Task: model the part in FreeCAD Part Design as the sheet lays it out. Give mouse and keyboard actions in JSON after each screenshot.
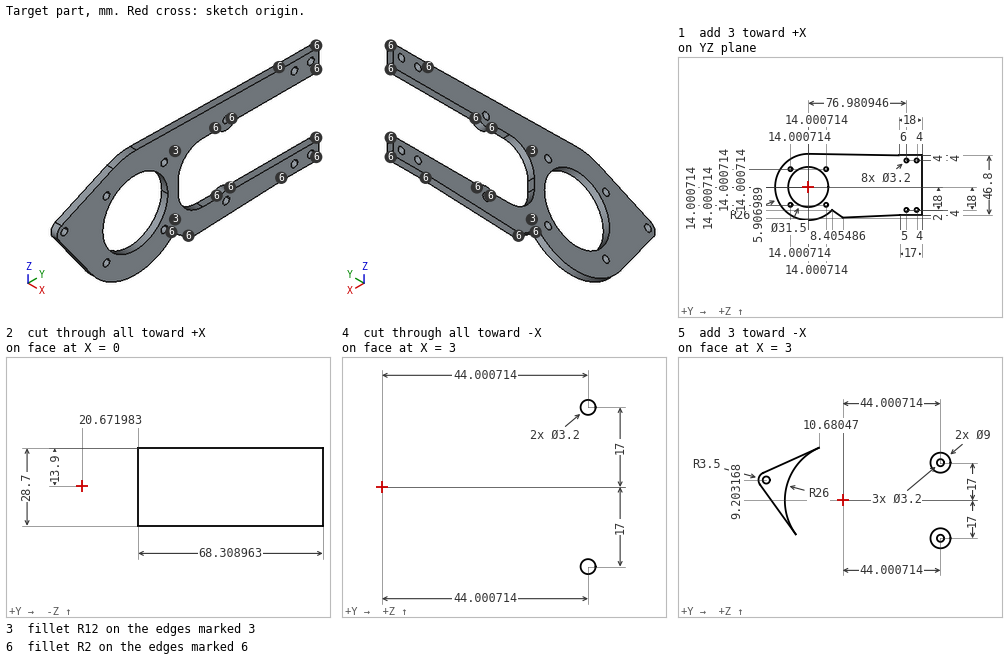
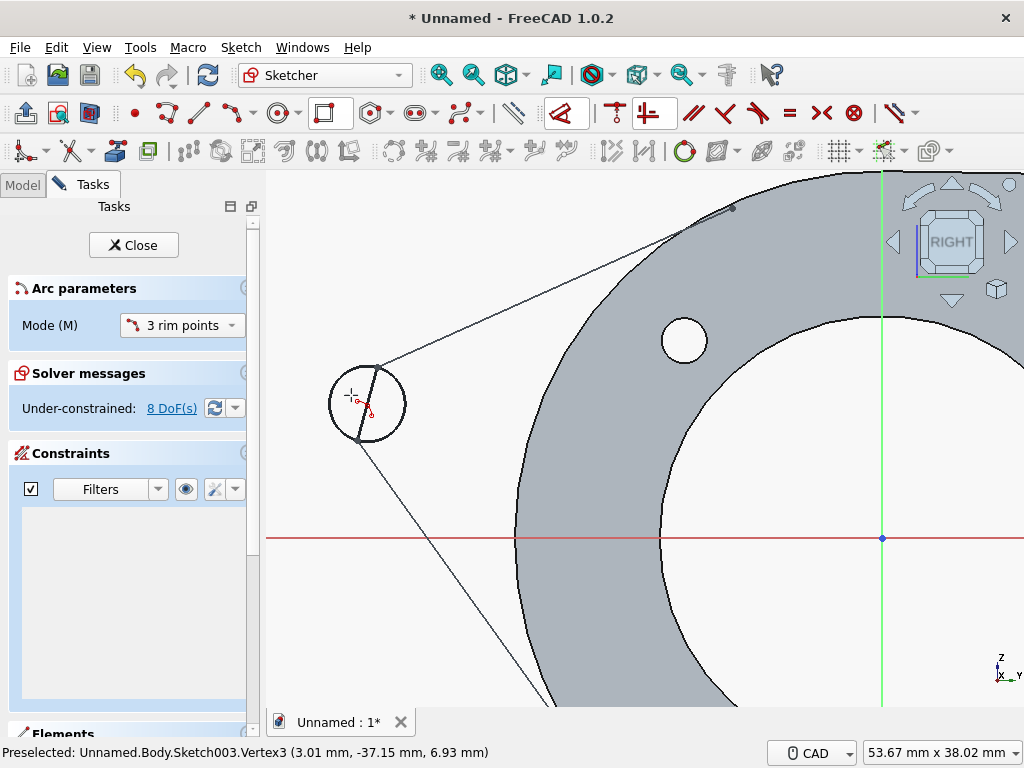
{"action": "left_click", "coordinate": [349, 396]}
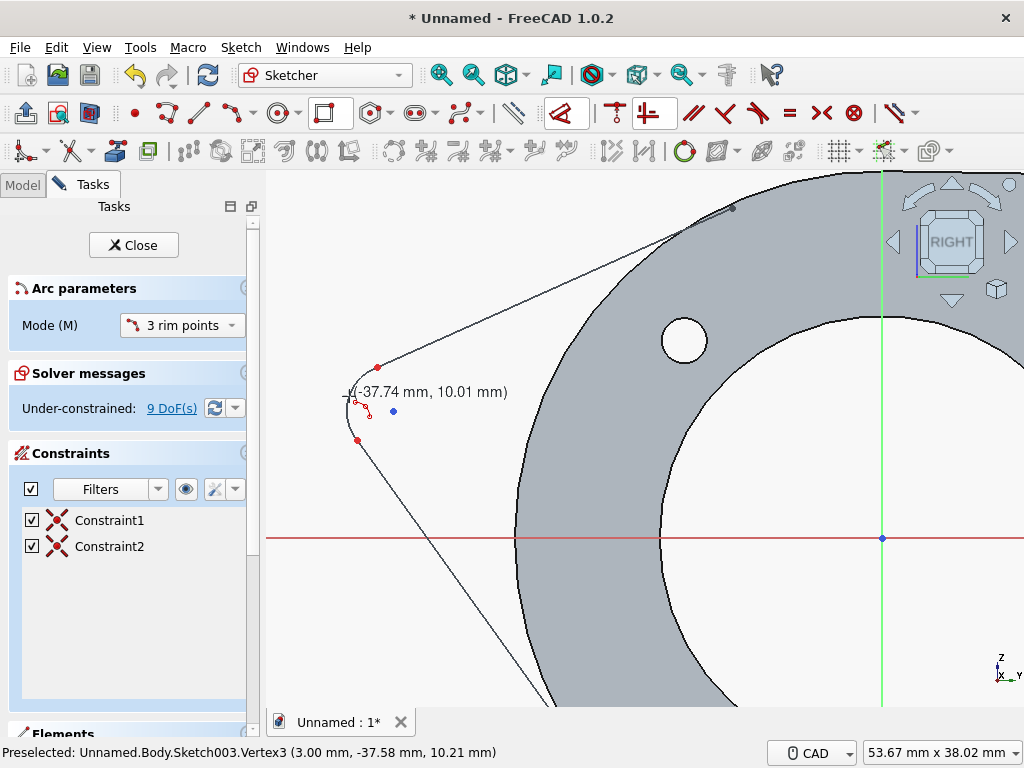
{"action": "scroll", "coordinate": [412, 402], "scroll_direction": "down", "scroll_amount": 6}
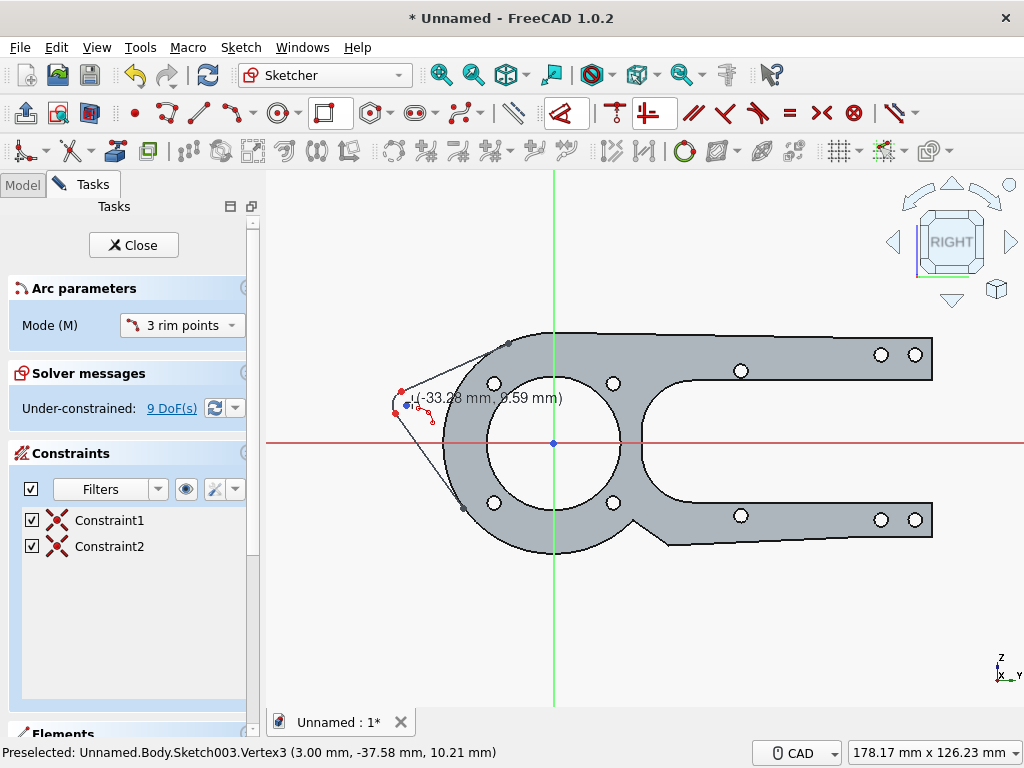
{"action": "left_click", "coordinate": [464, 509]}
{"action": "left_click", "coordinate": [509, 344]}
{"action": "left_click", "coordinate": [447, 415]}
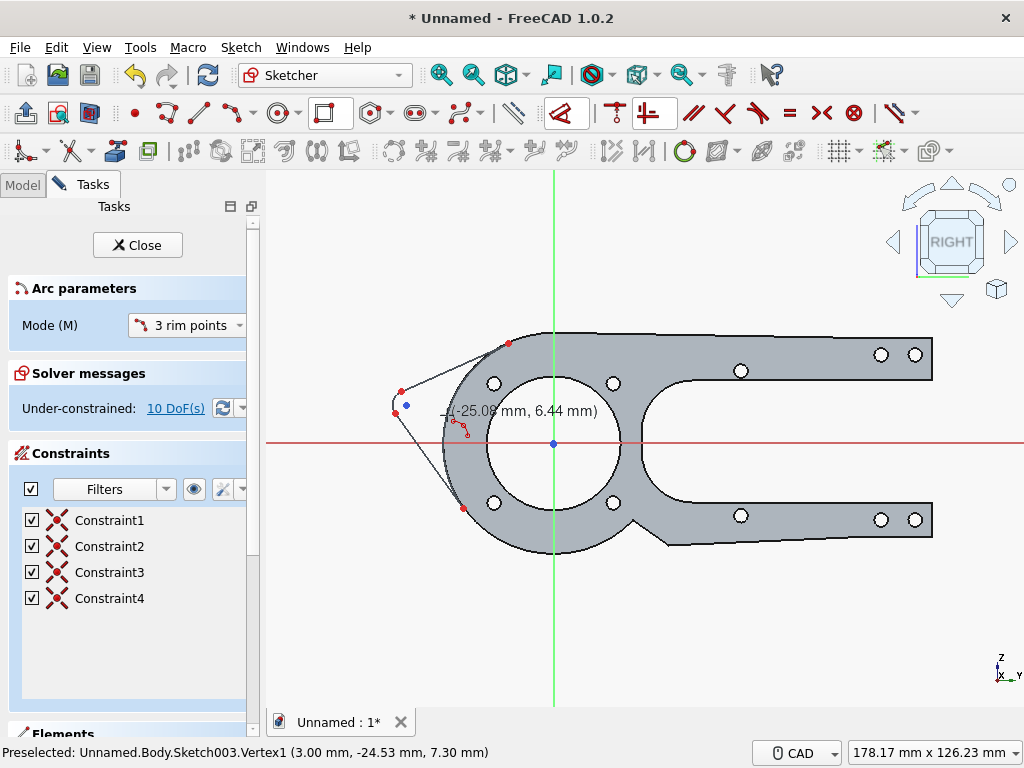
{"action": "left_click", "coordinate": [278, 114]}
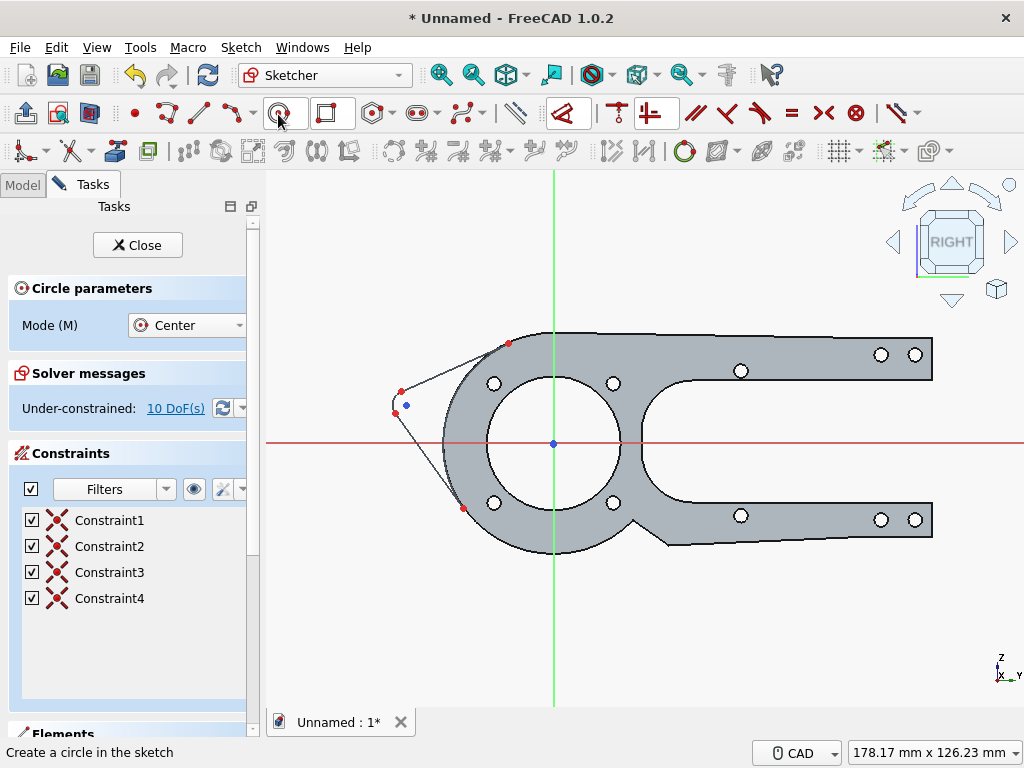
{"action": "left_click", "coordinate": [741, 371]}
{"action": "left_click", "coordinate": [754, 358]}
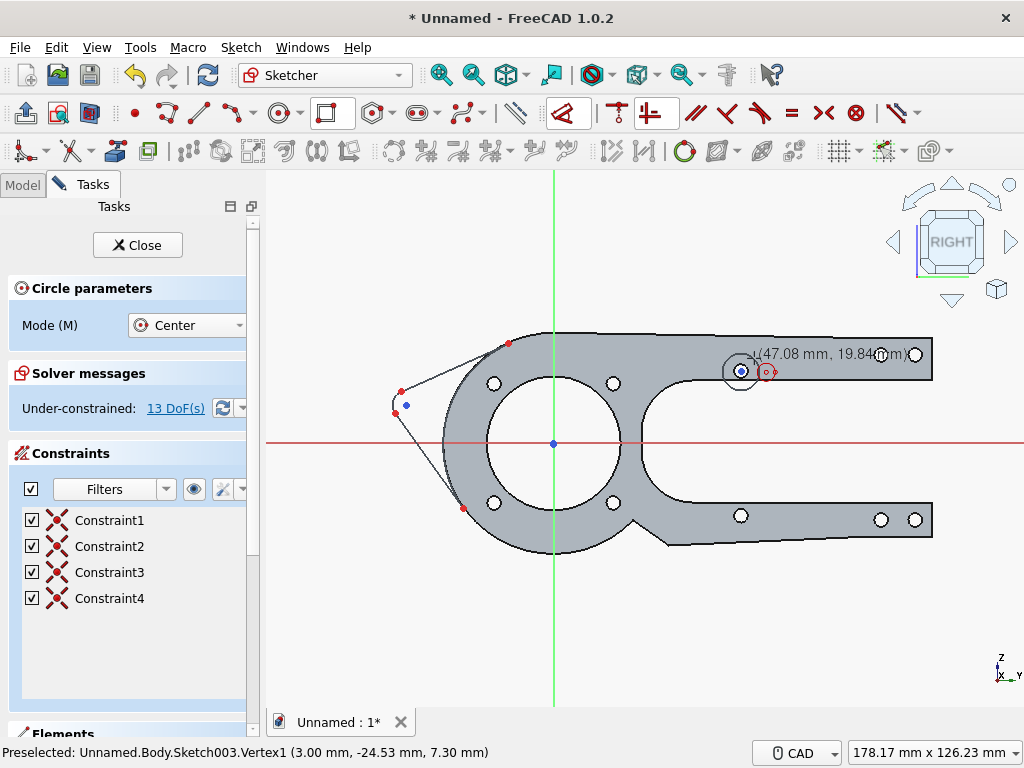
{"action": "left_click", "coordinate": [741, 516]}
{"action": "left_click", "coordinate": [754, 502]}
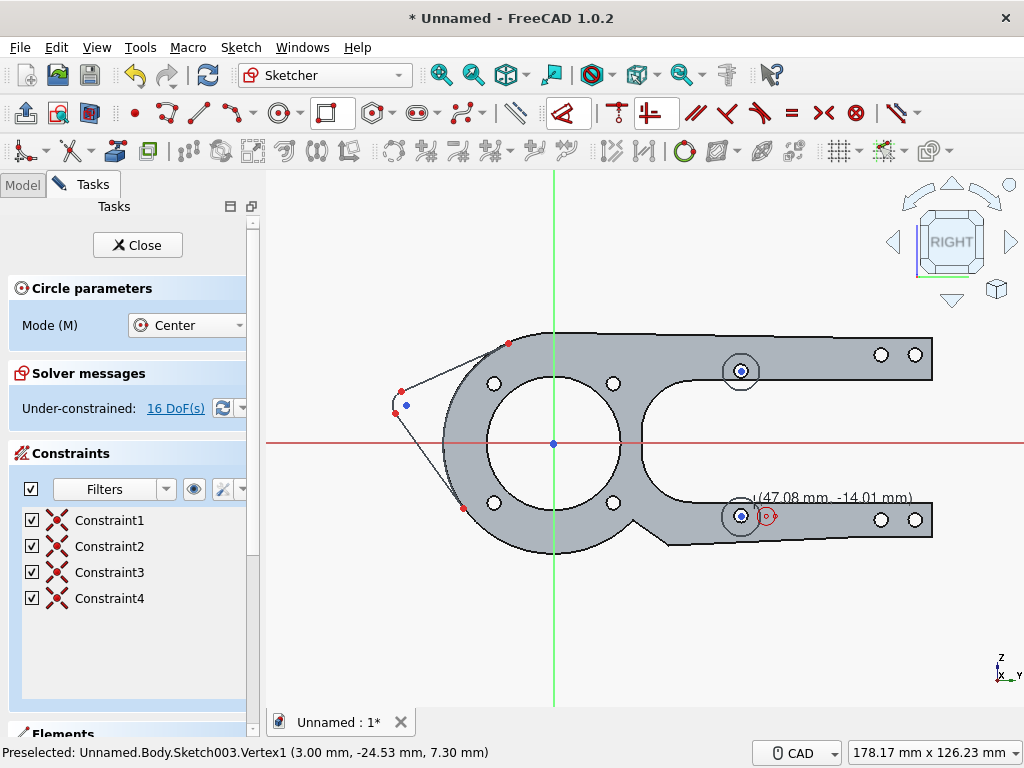
{"action": "scroll", "coordinate": [741, 371], "scroll_direction": "up", "scroll_amount": 7}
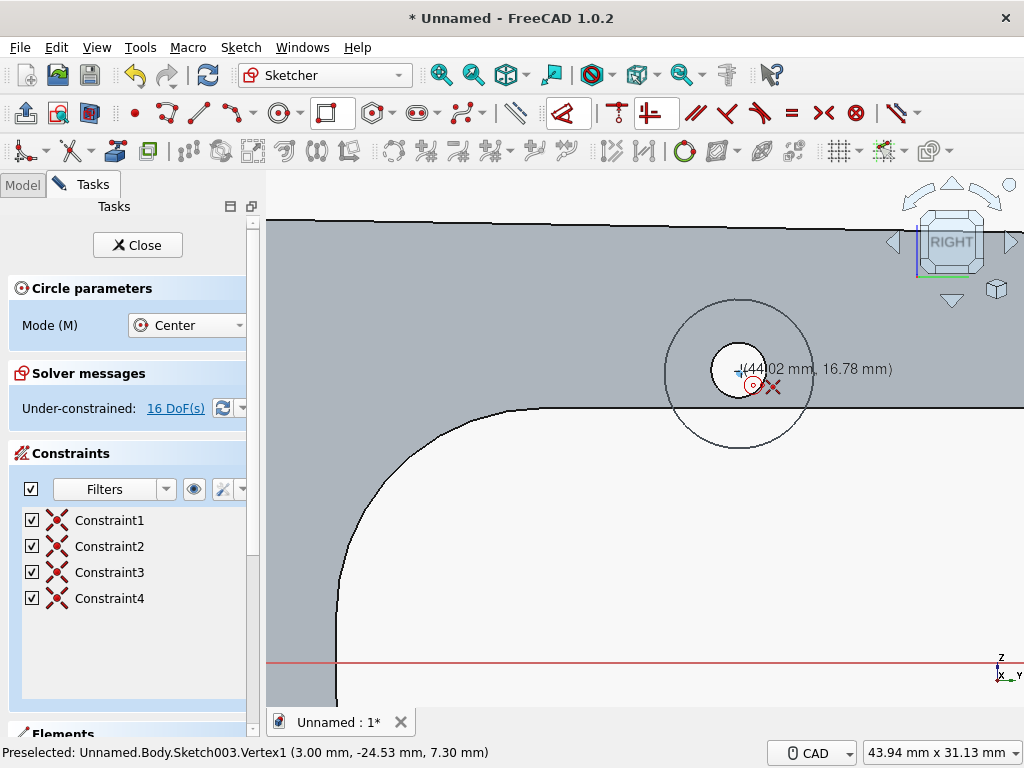
{"action": "scroll", "coordinate": [741, 371], "scroll_direction": "down", "scroll_amount": 7}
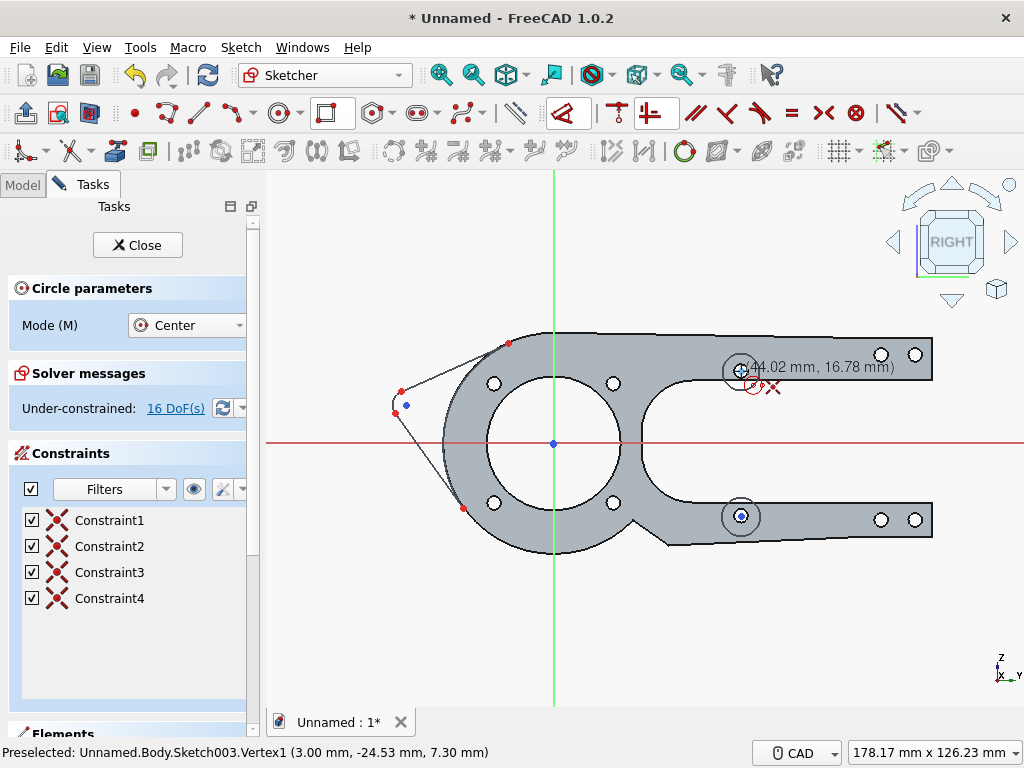
{"action": "left_click", "coordinate": [741, 372]}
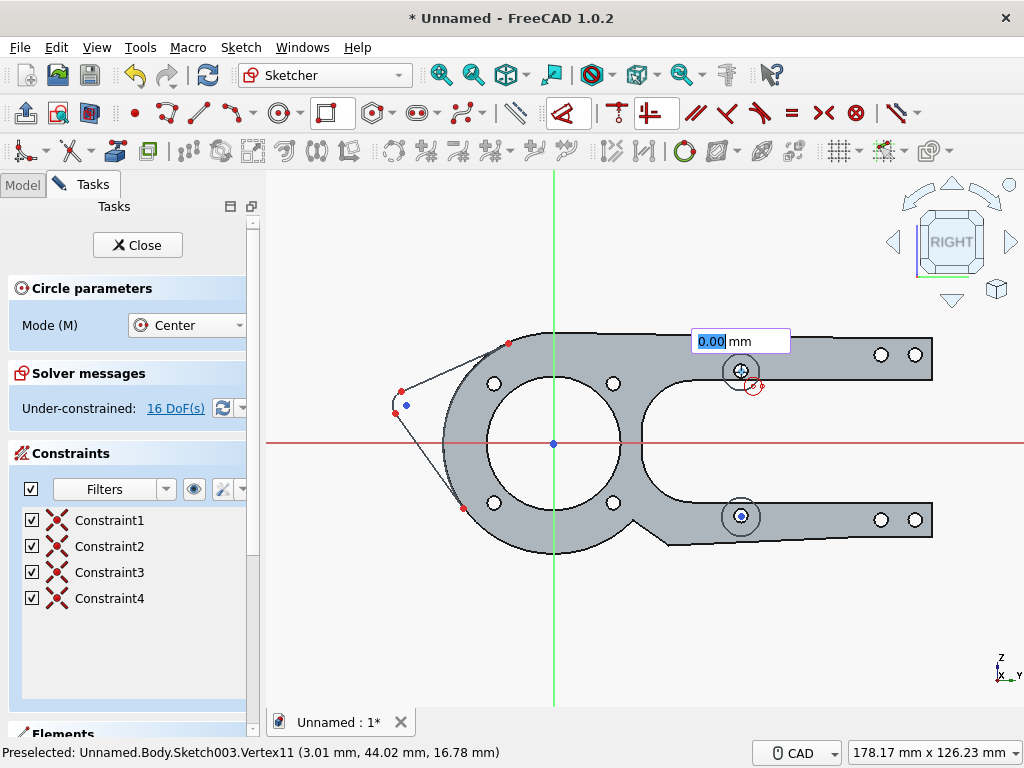
{"action": "scroll", "coordinate": [747, 369], "scroll_direction": "up", "scroll_amount": 5}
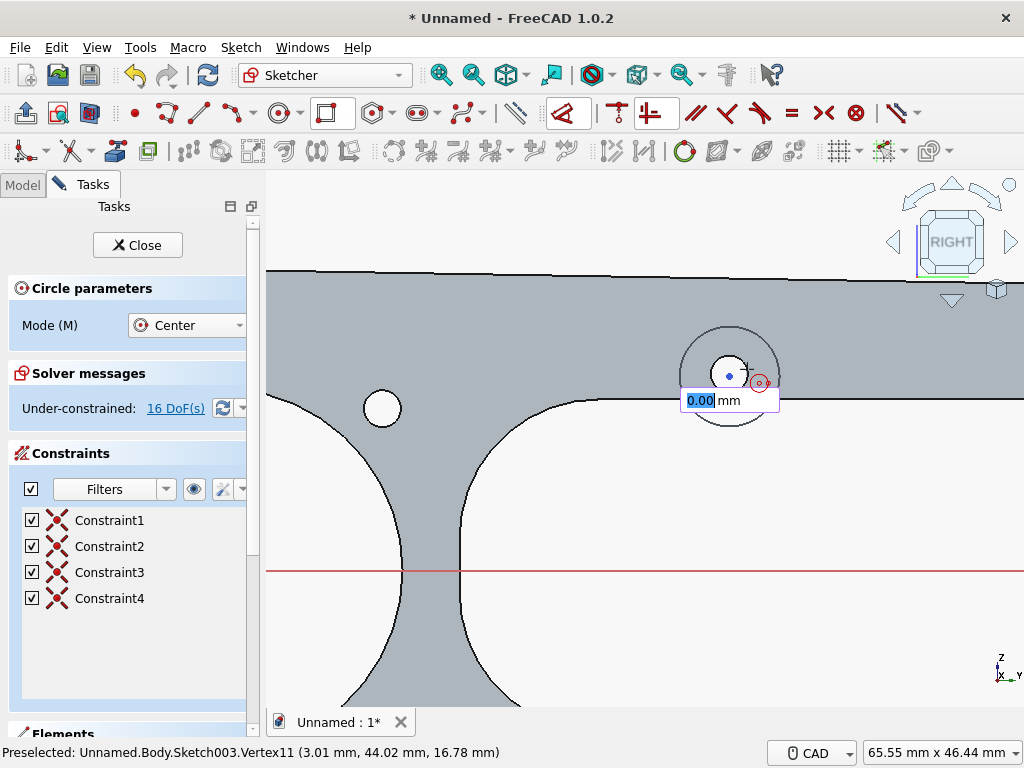
{"action": "left_click", "coordinate": [747, 368]}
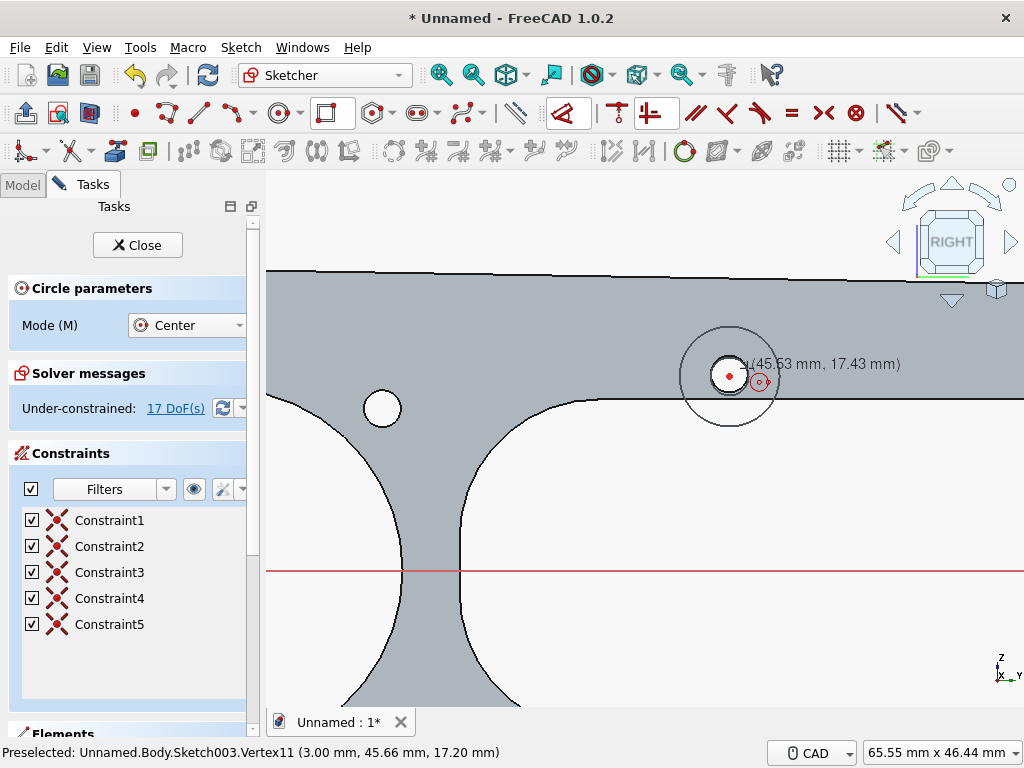
{"action": "scroll", "coordinate": [747, 369], "scroll_direction": "down", "scroll_amount": 5}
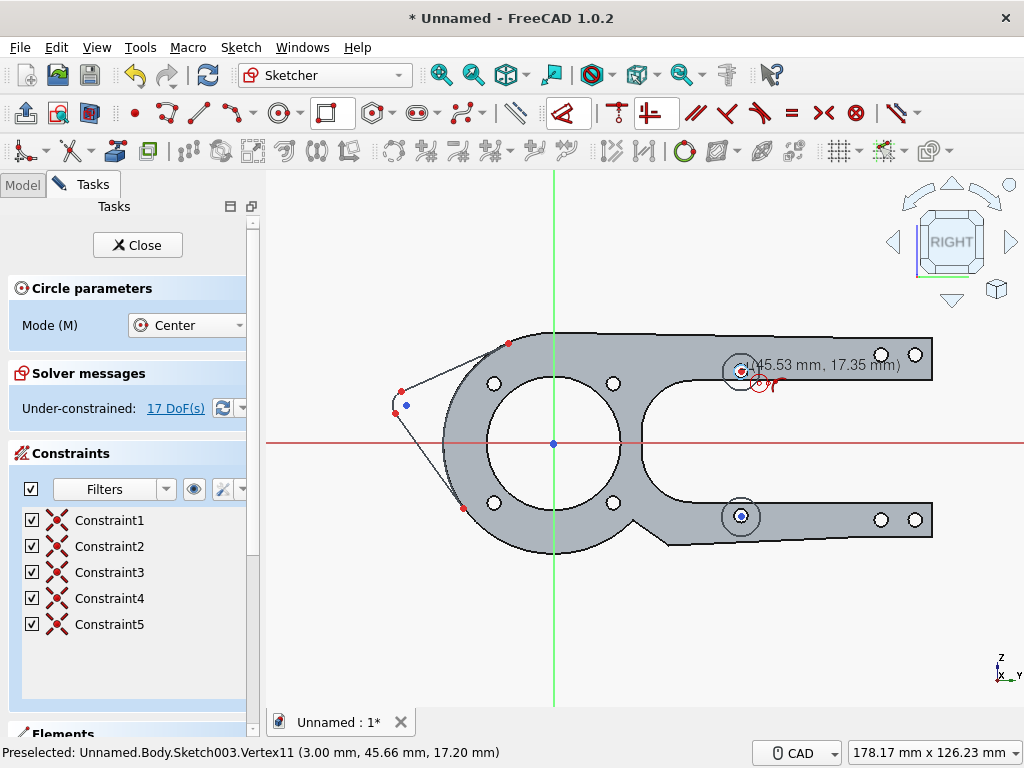
{"action": "scroll", "coordinate": [741, 516], "scroll_direction": "up", "scroll_amount": 7}